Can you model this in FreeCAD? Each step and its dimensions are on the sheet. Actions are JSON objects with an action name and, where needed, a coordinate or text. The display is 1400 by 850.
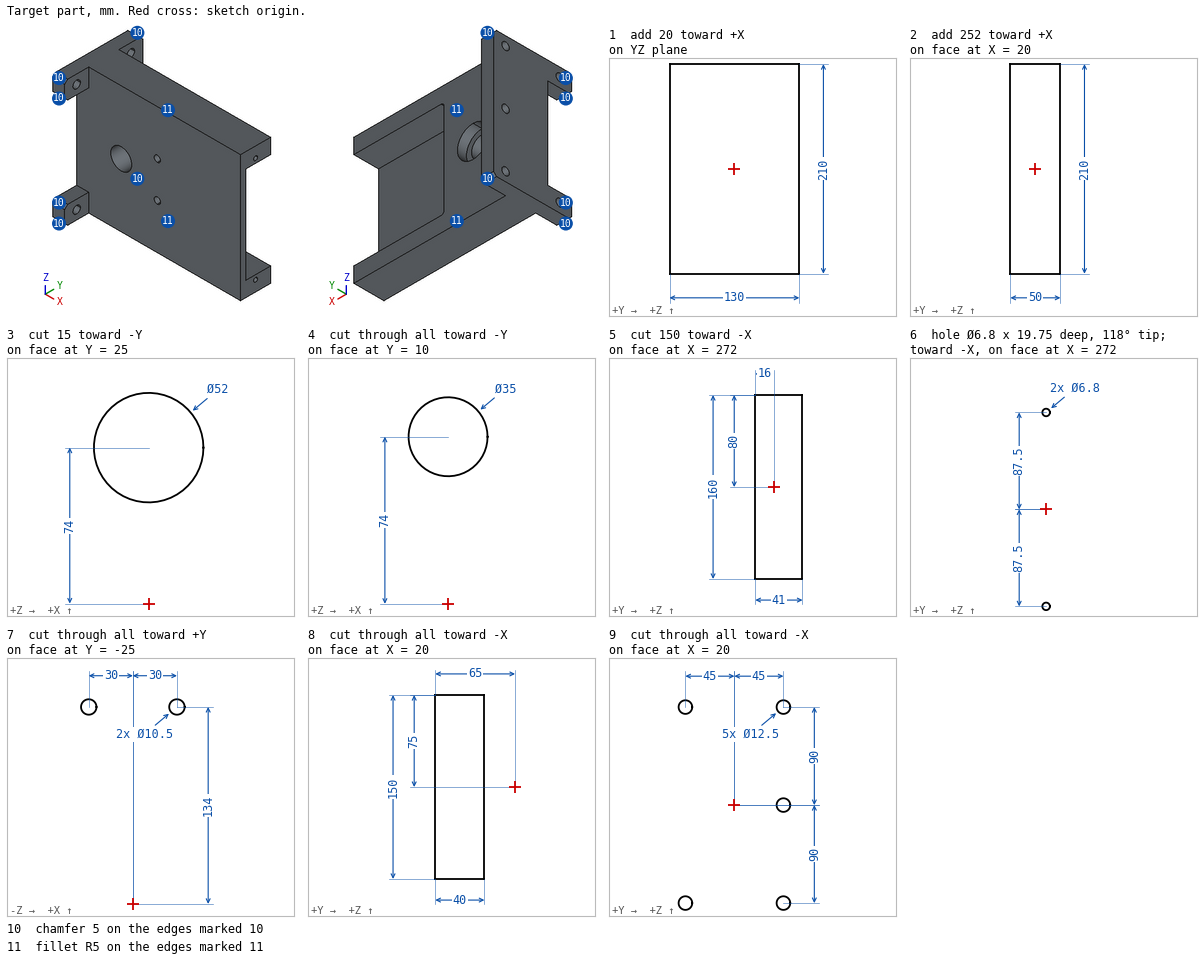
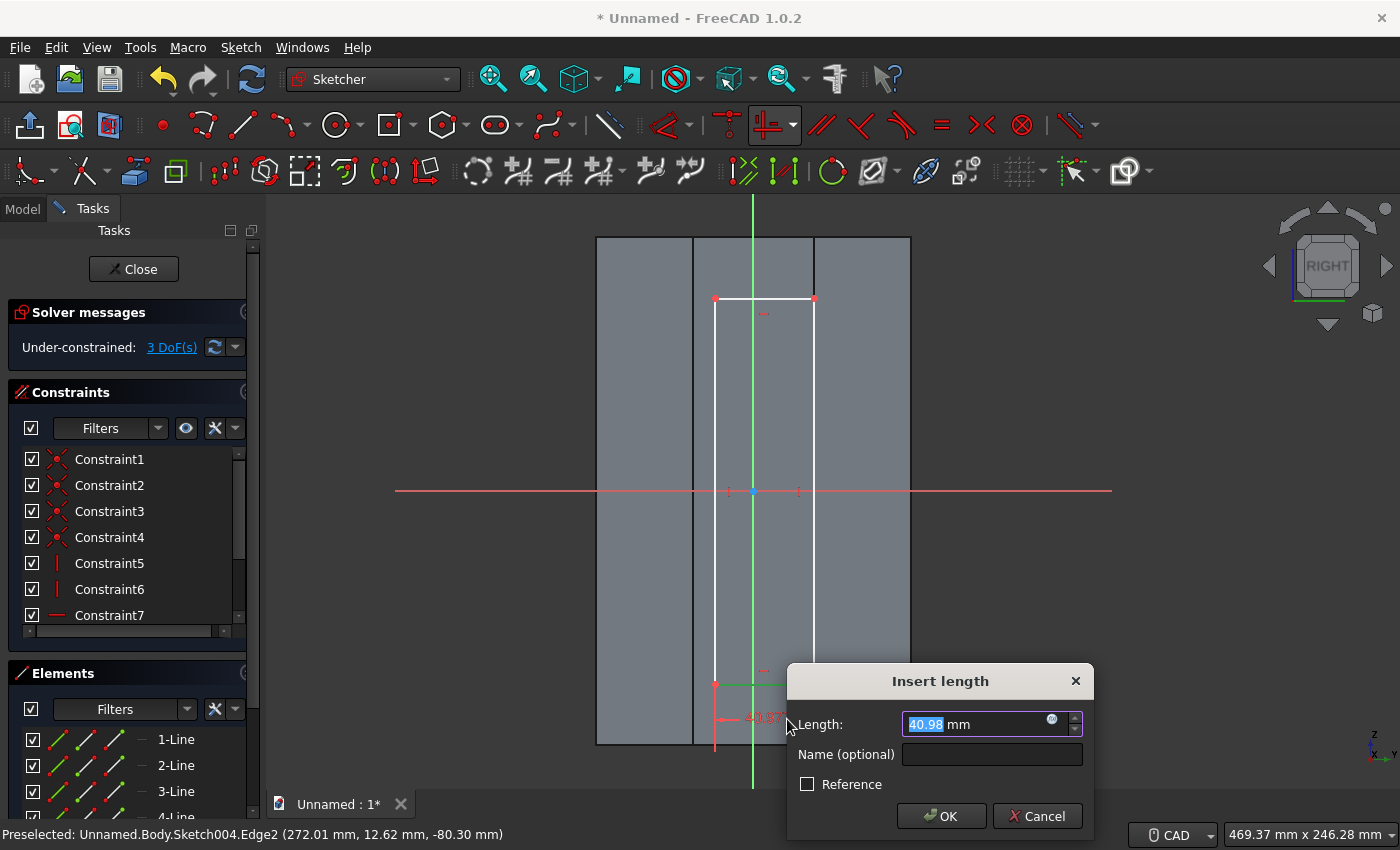
{"action": "type", "text": "41"}
{"action": "key", "text": "Return"}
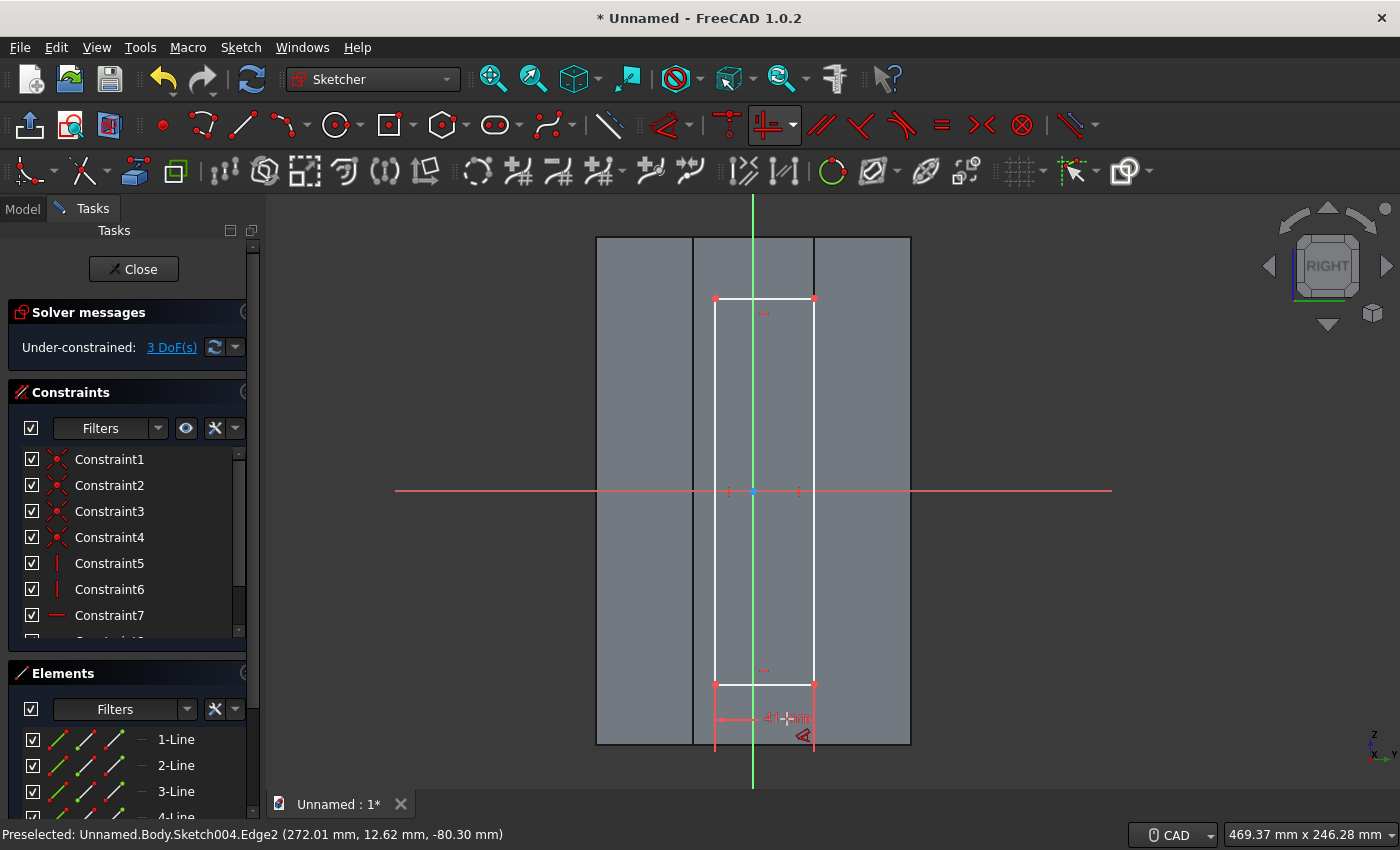
{"action": "left_click", "coordinate": [715, 415]}
{"action": "left_click", "coordinate": [681, 403]}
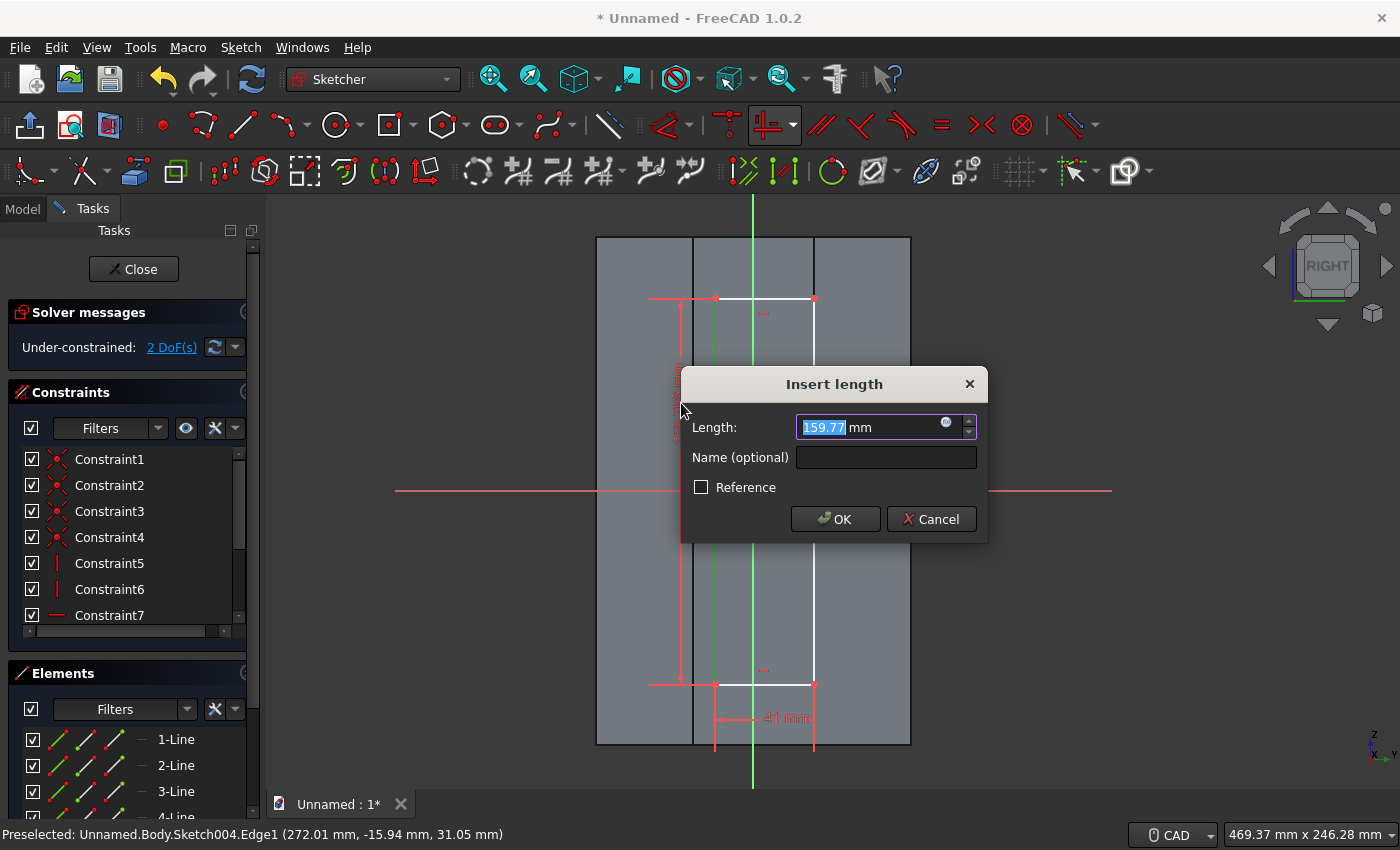
{"action": "type", "text": "160"}
{"action": "key", "text": "Return"}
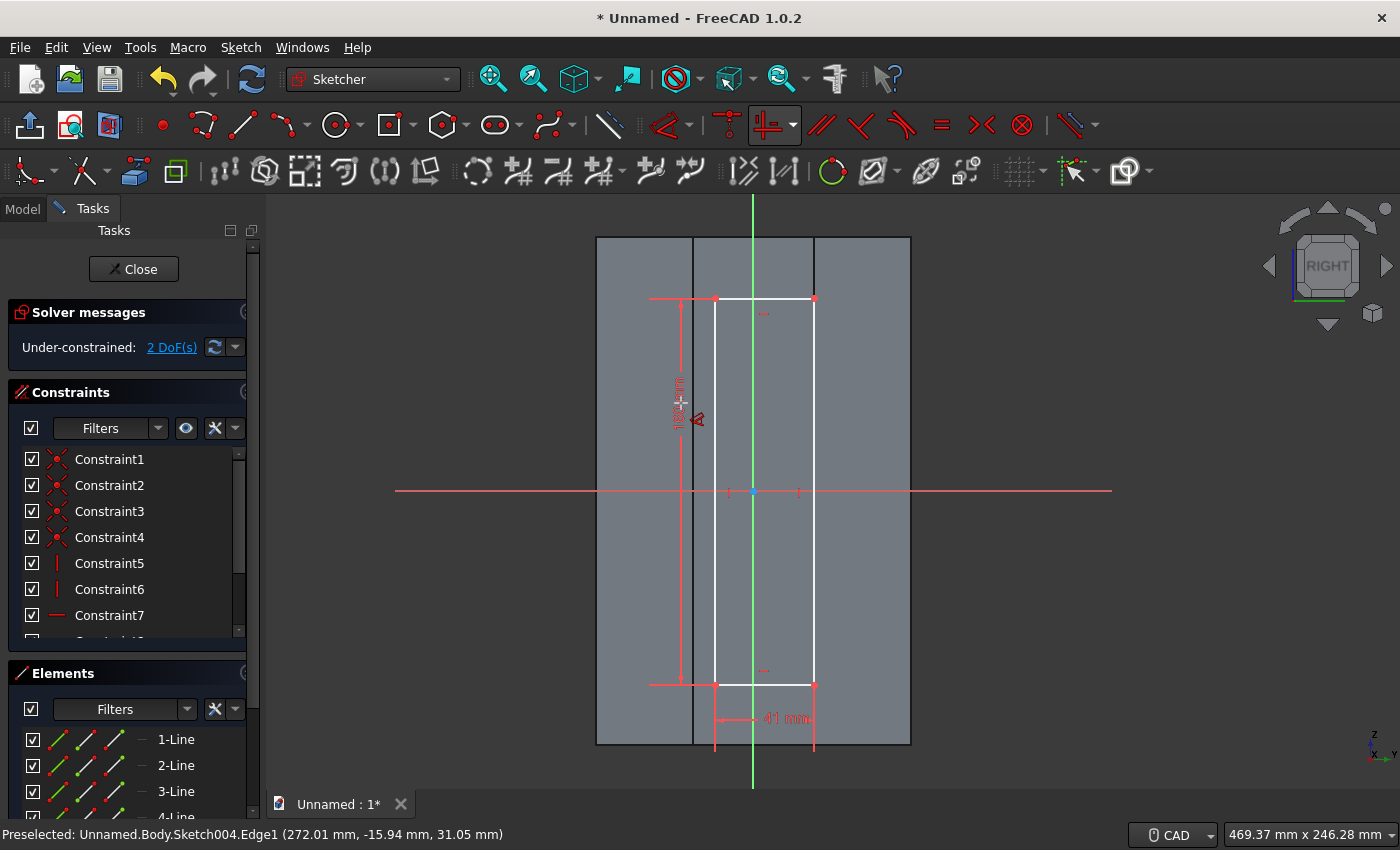
{"action": "left_click", "coordinate": [715, 299]}
{"action": "left_click", "coordinate": [734, 265]}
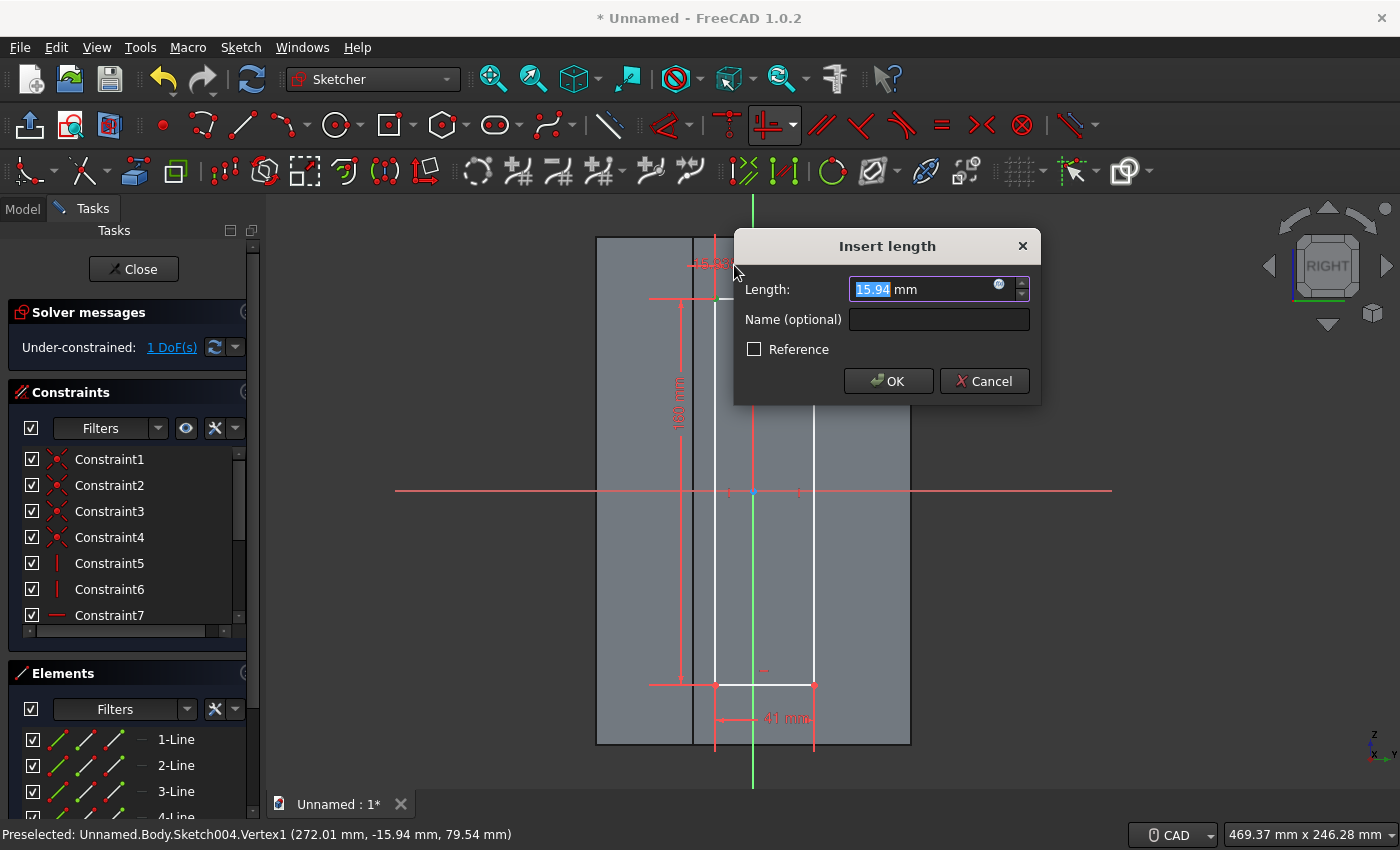
{"action": "type", "text": "16"}
{"action": "key", "text": "Return"}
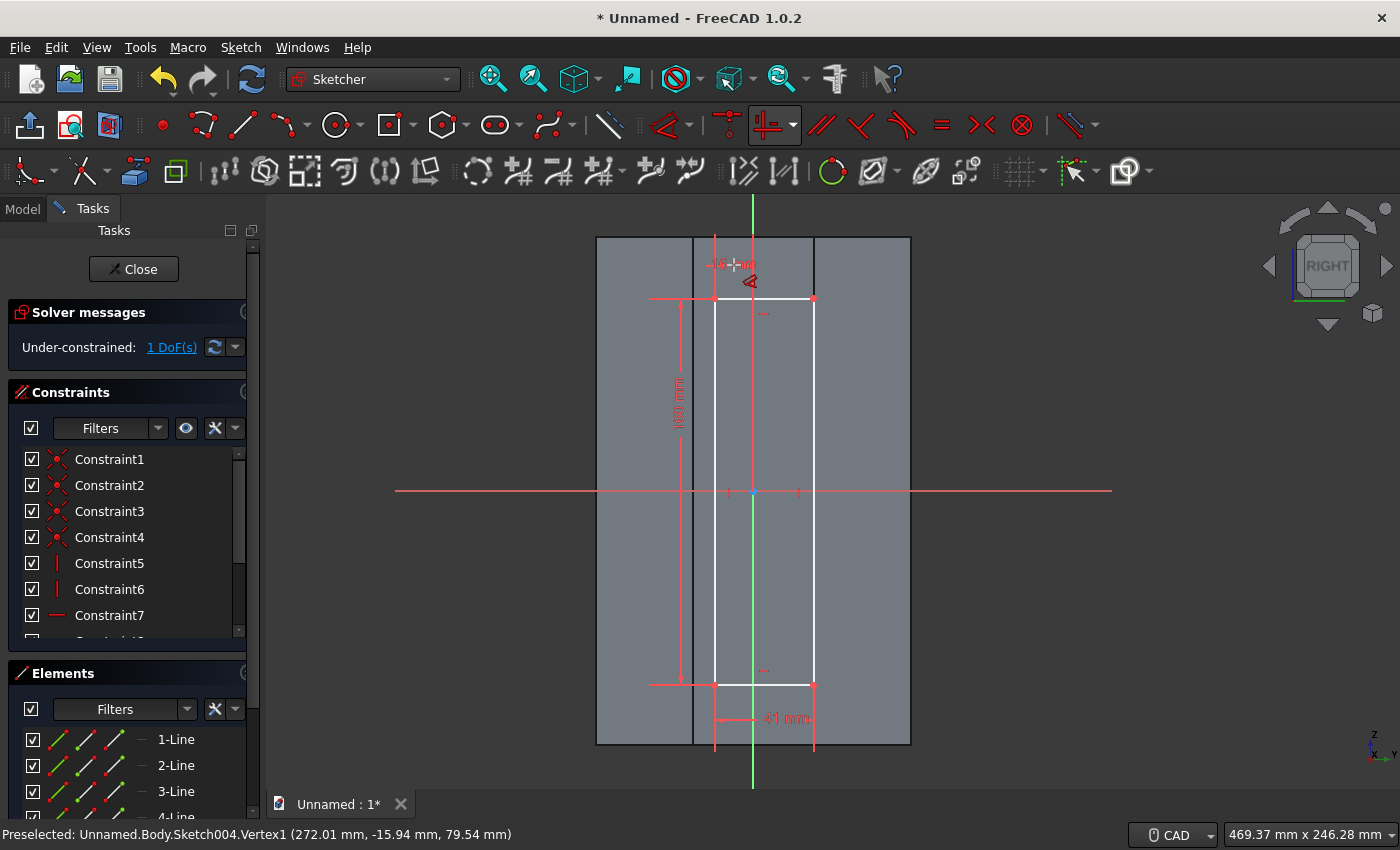
{"action": "left_click", "coordinate": [715, 299]}
{"action": "left_click", "coordinate": [681, 351]}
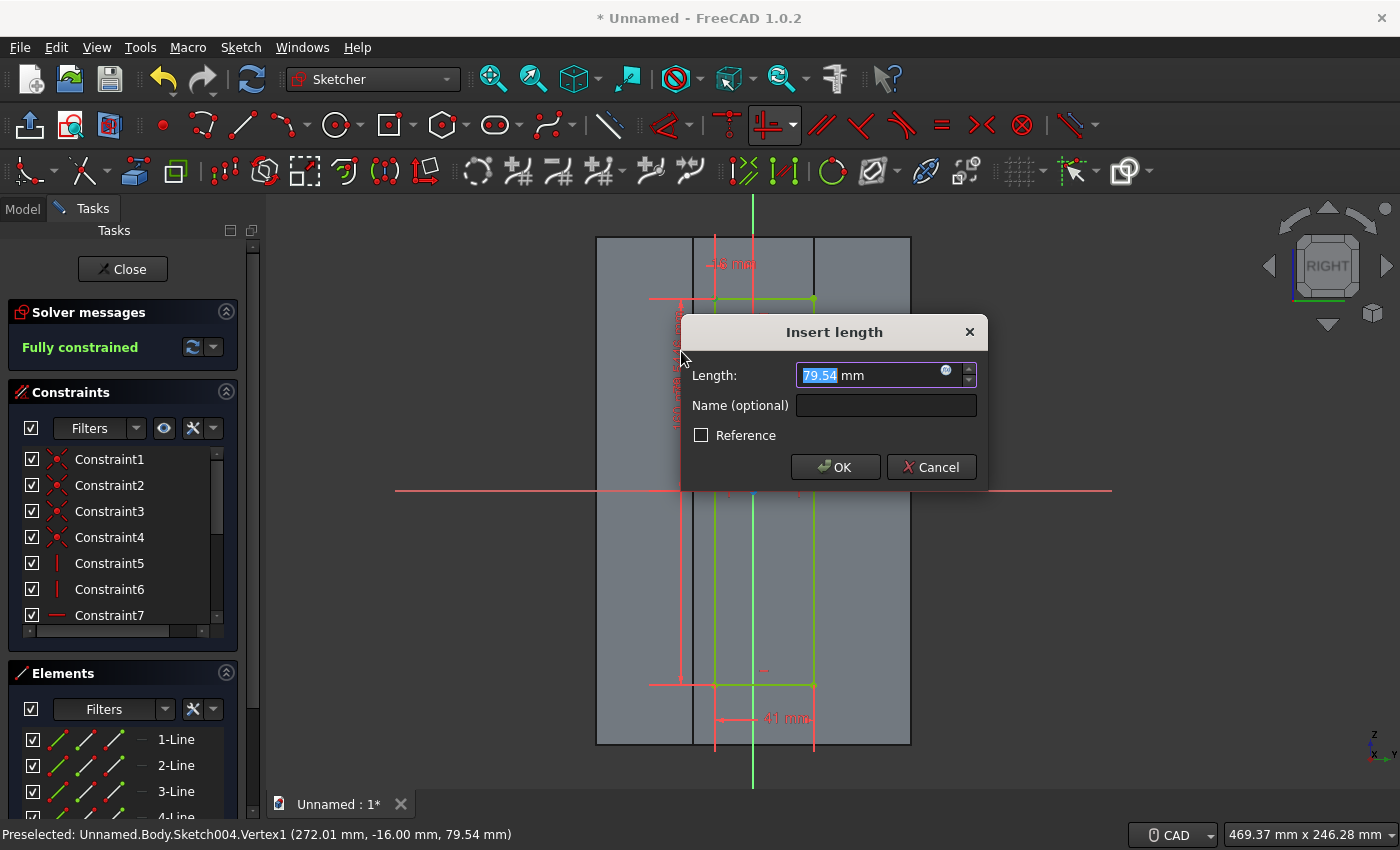
{"action": "type", "text": "80"}
{"action": "key", "text": "Return"}
{"action": "key", "text": "Escape"}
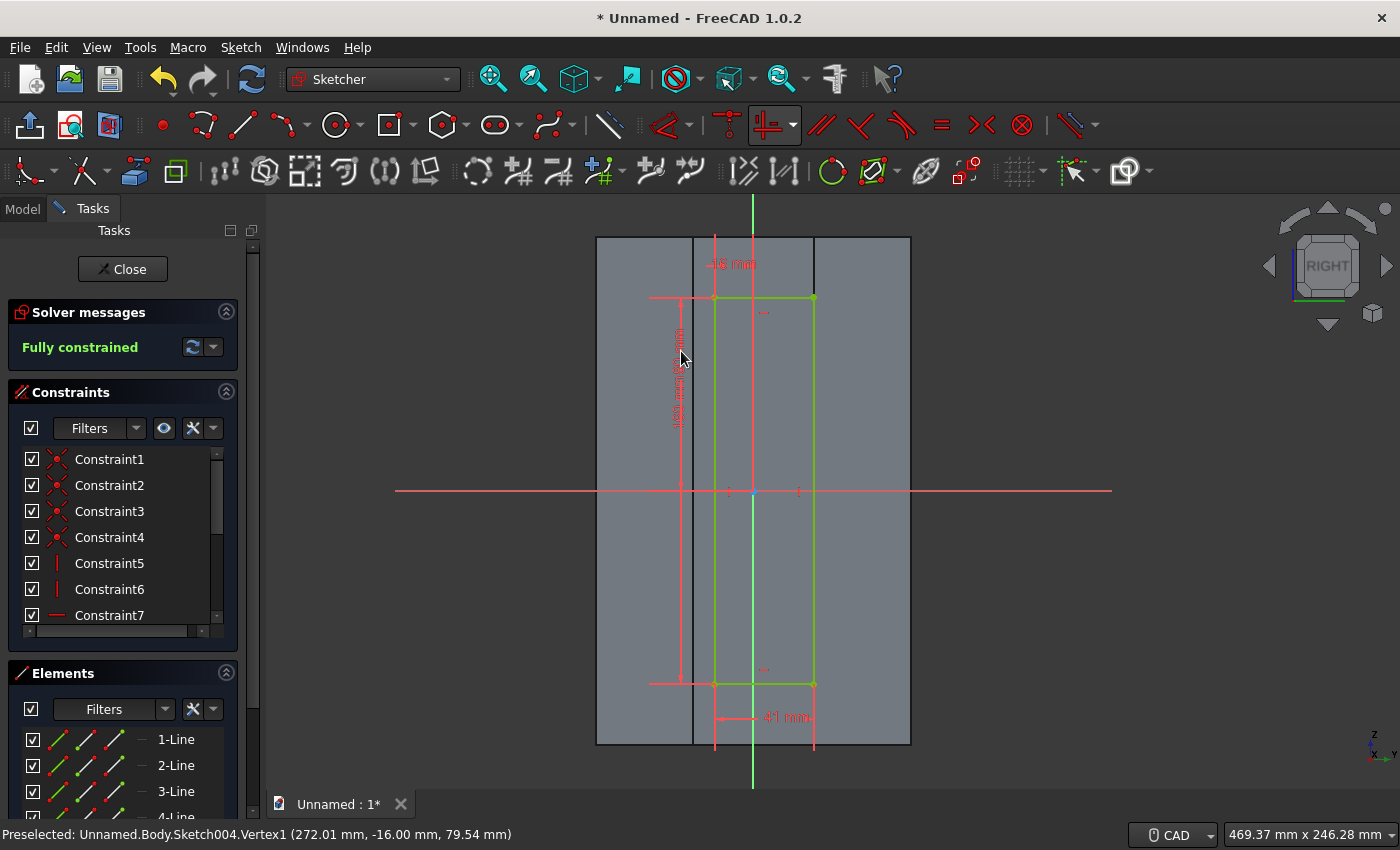
{"action": "left_click", "coordinate": [123, 269]}